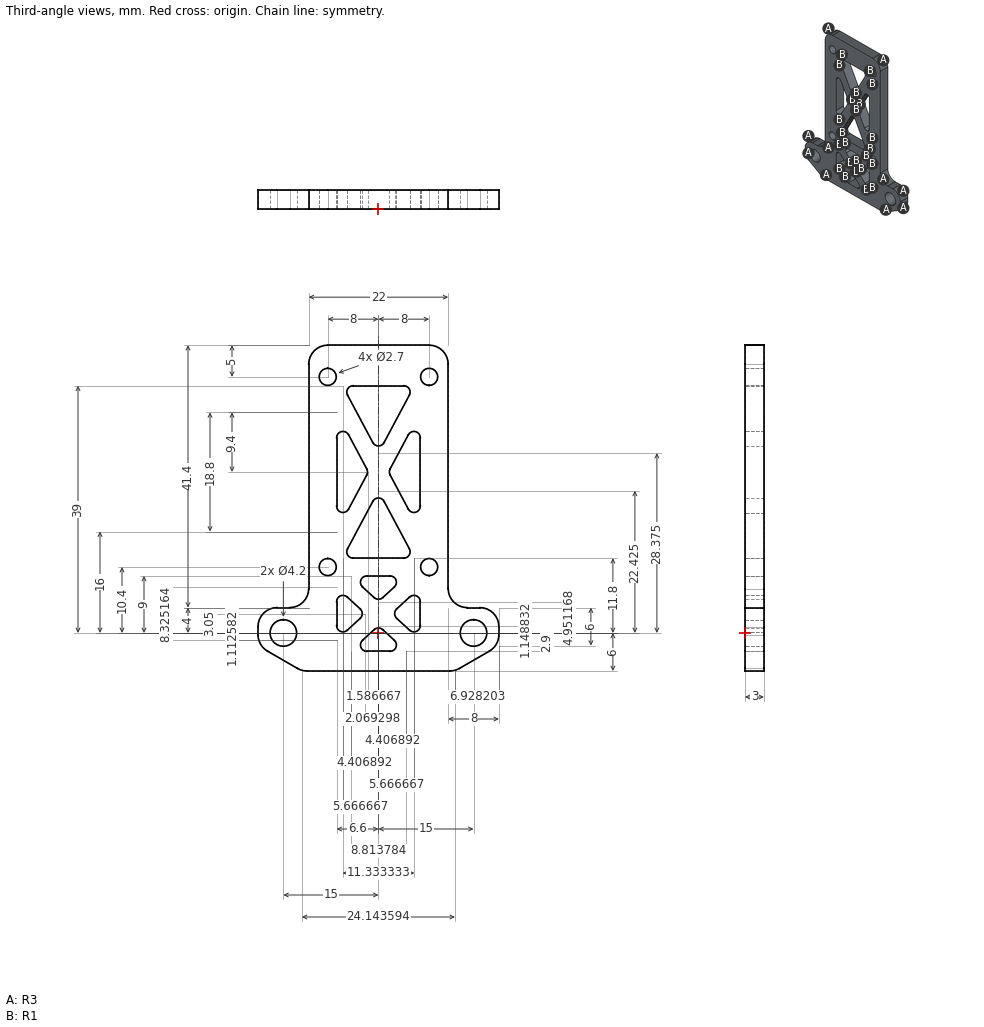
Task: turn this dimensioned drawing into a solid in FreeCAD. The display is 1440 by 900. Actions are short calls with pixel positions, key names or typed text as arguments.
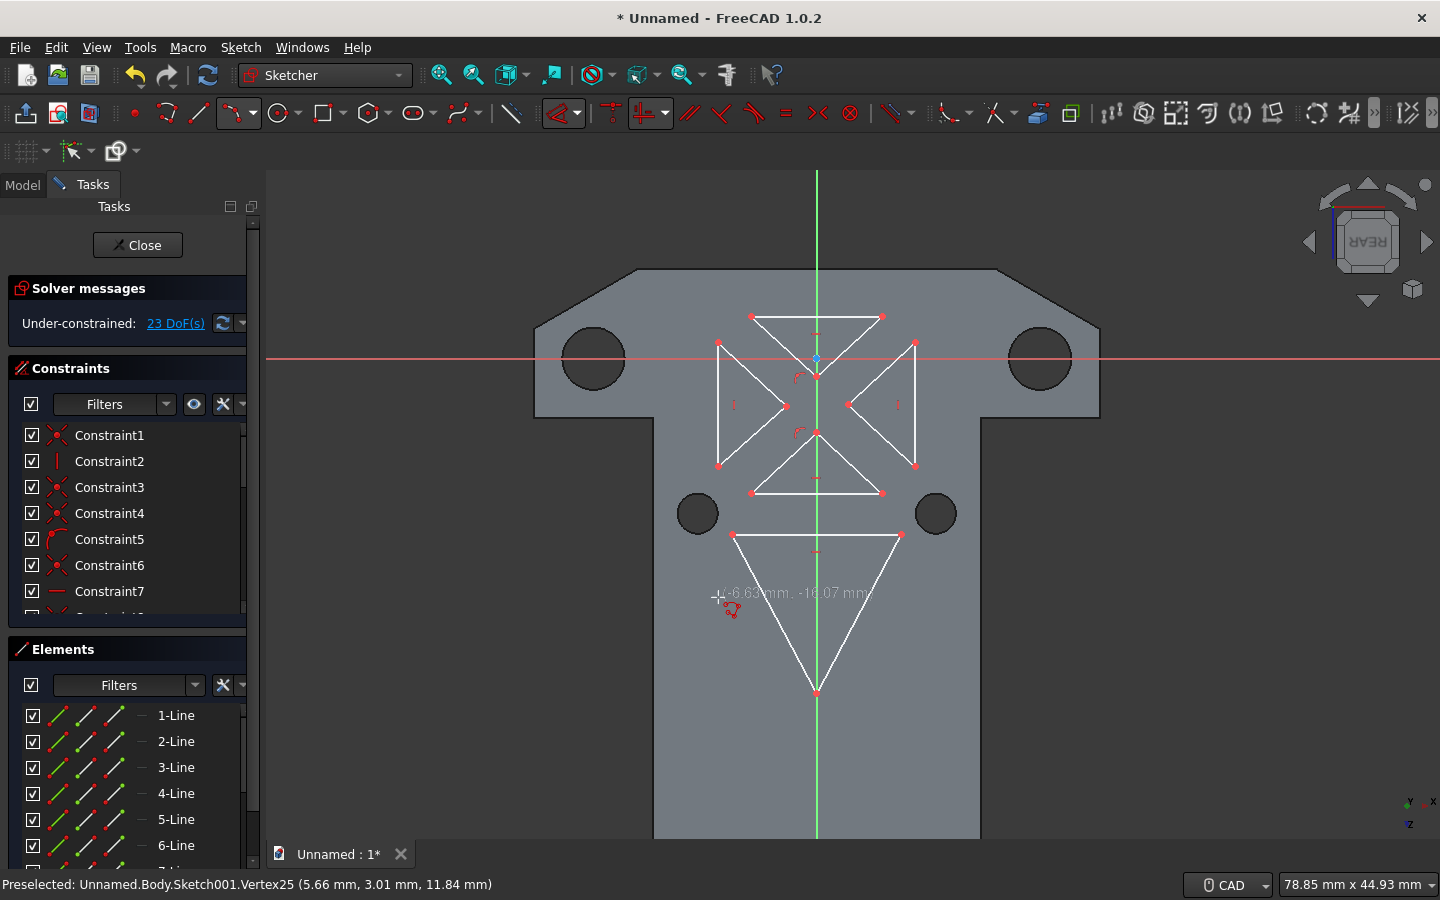
scroll(719, 255, down, 2)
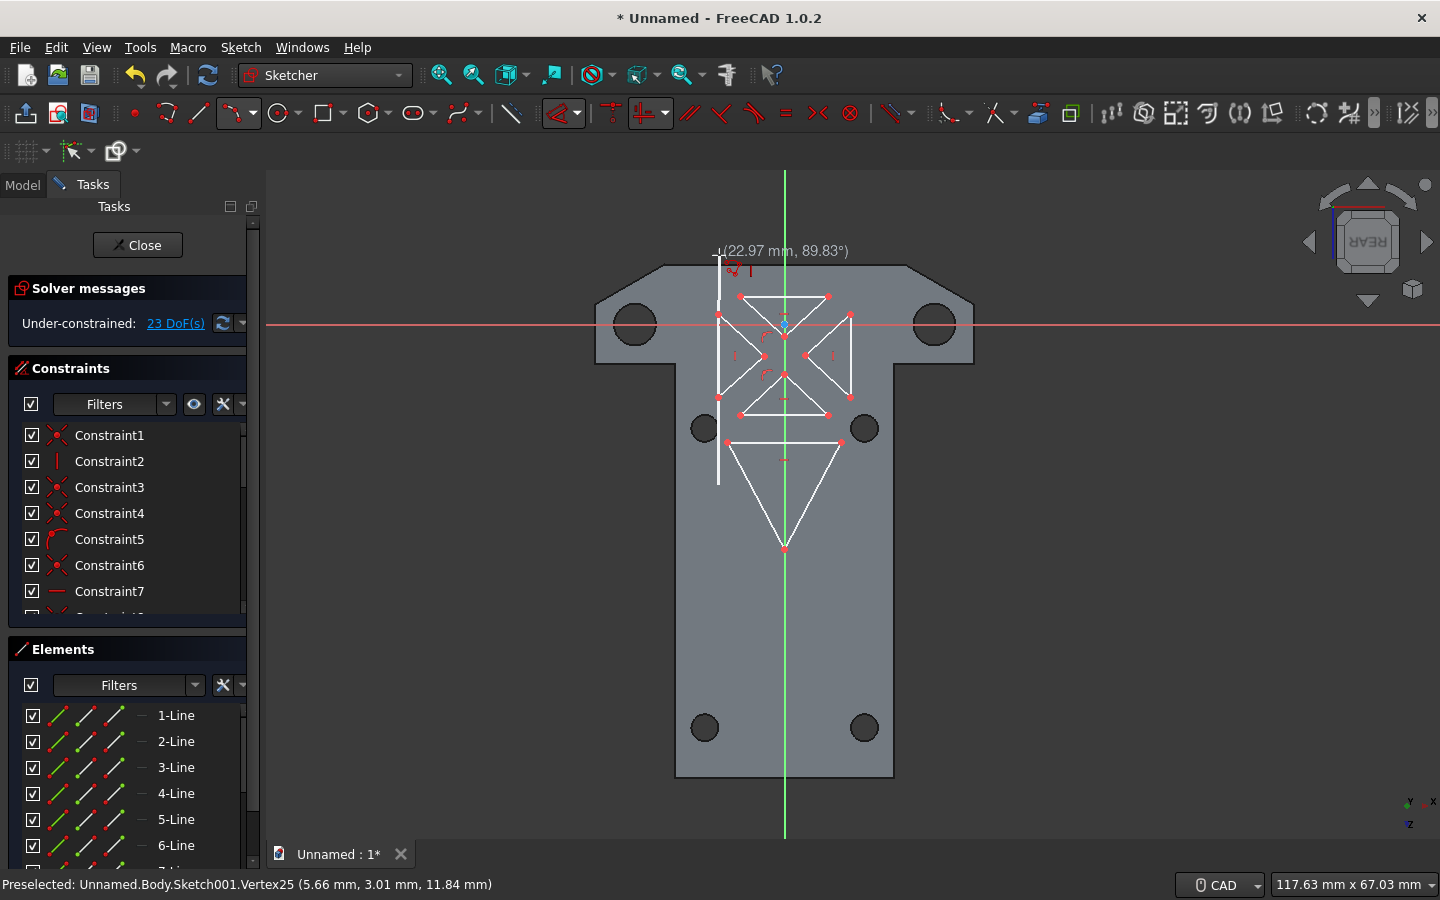
click(718, 672)
click(769, 578)
click(718, 485)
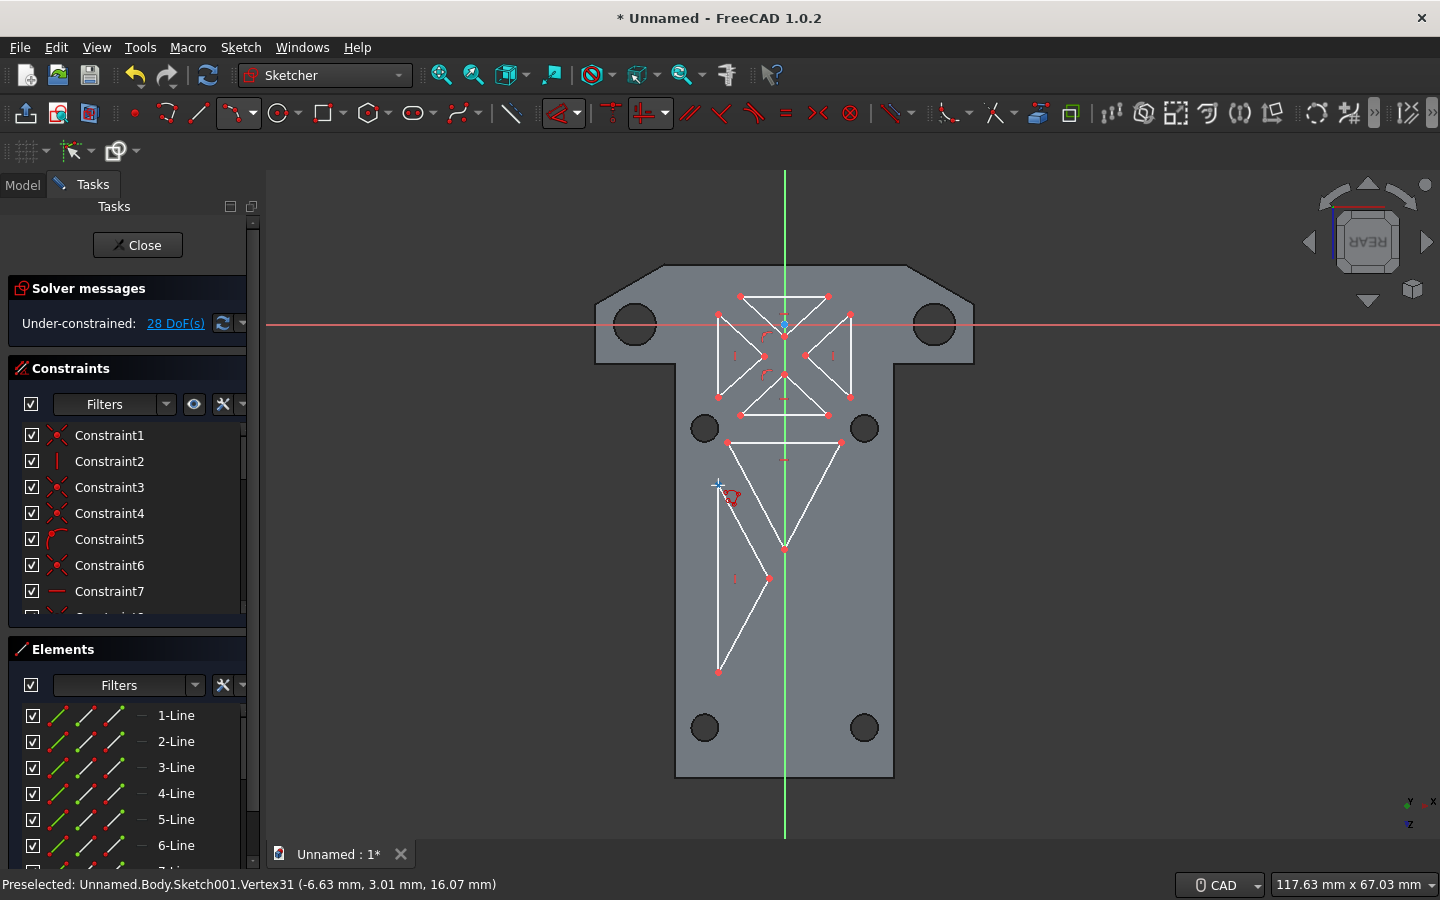
click(785, 608)
click(728, 714)
click(841, 714)
click(785, 609)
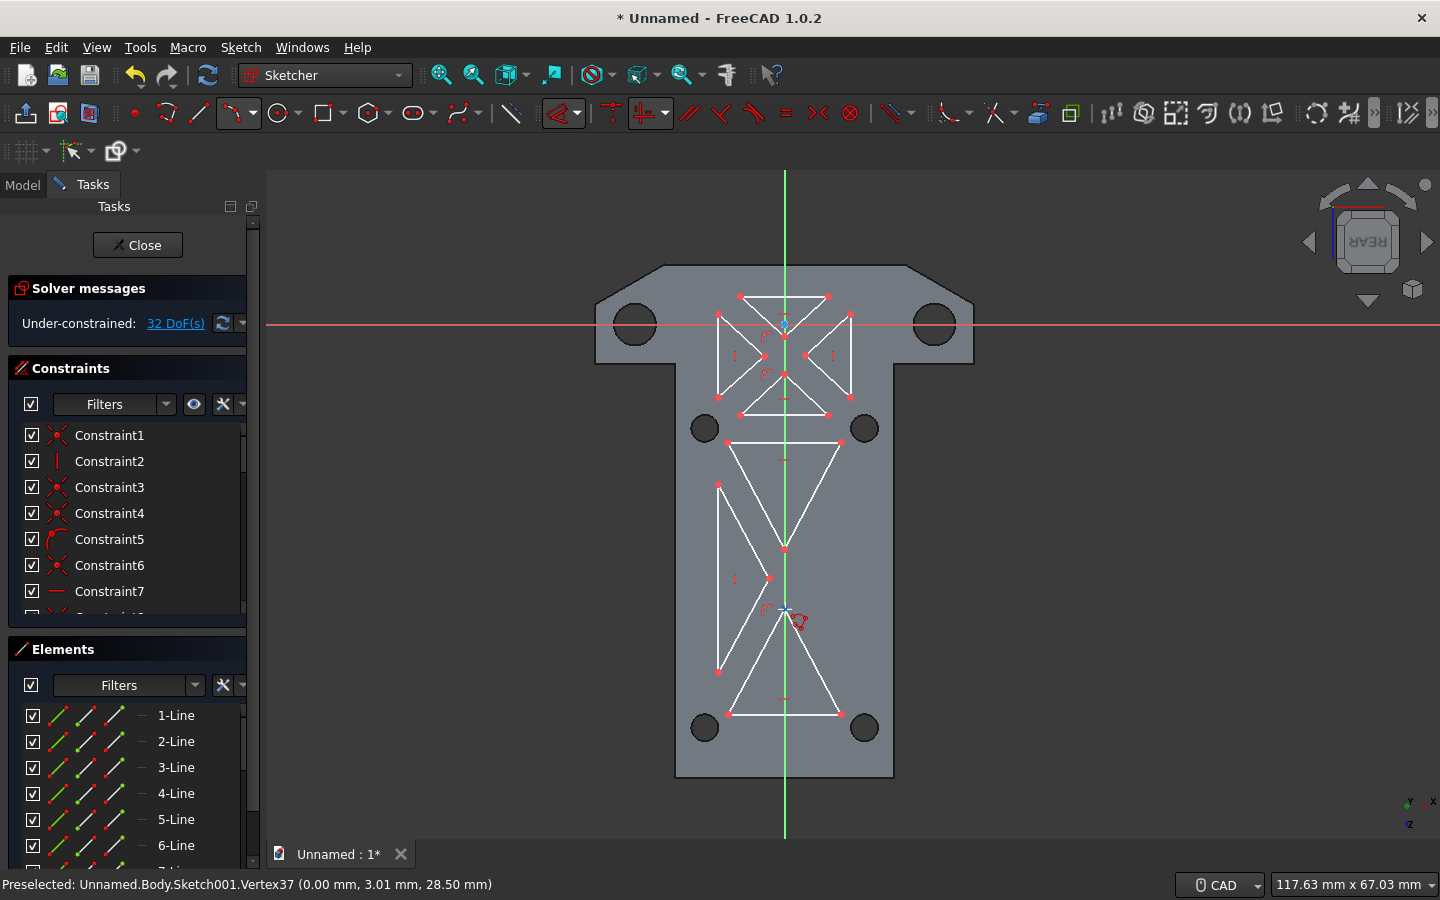
click(851, 484)
click(800, 578)
click(851, 672)
click(851, 485)
key(Escape)
key(Escape)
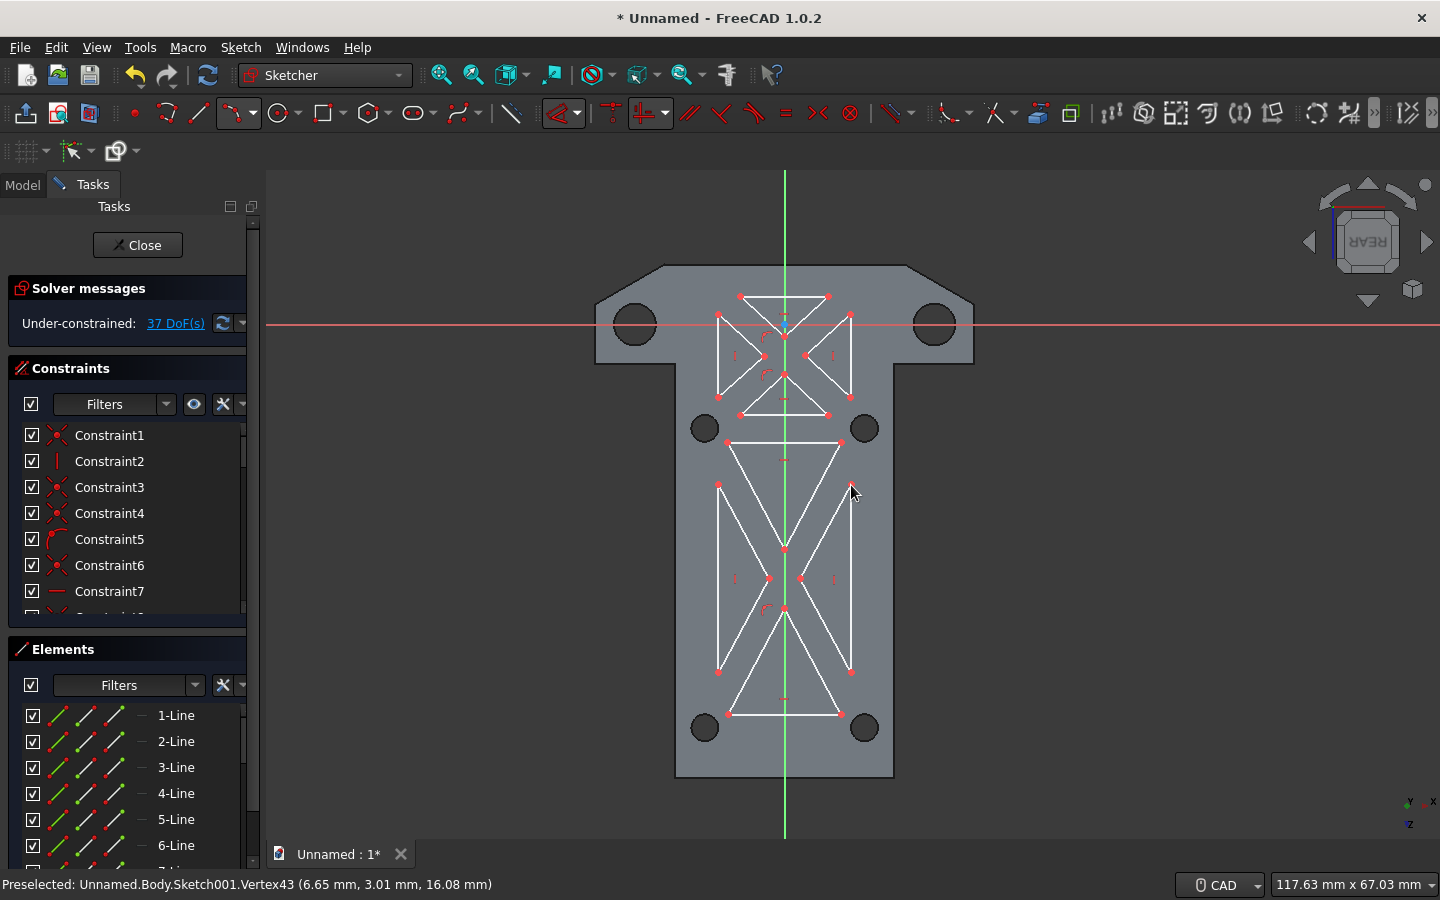
click(764, 356)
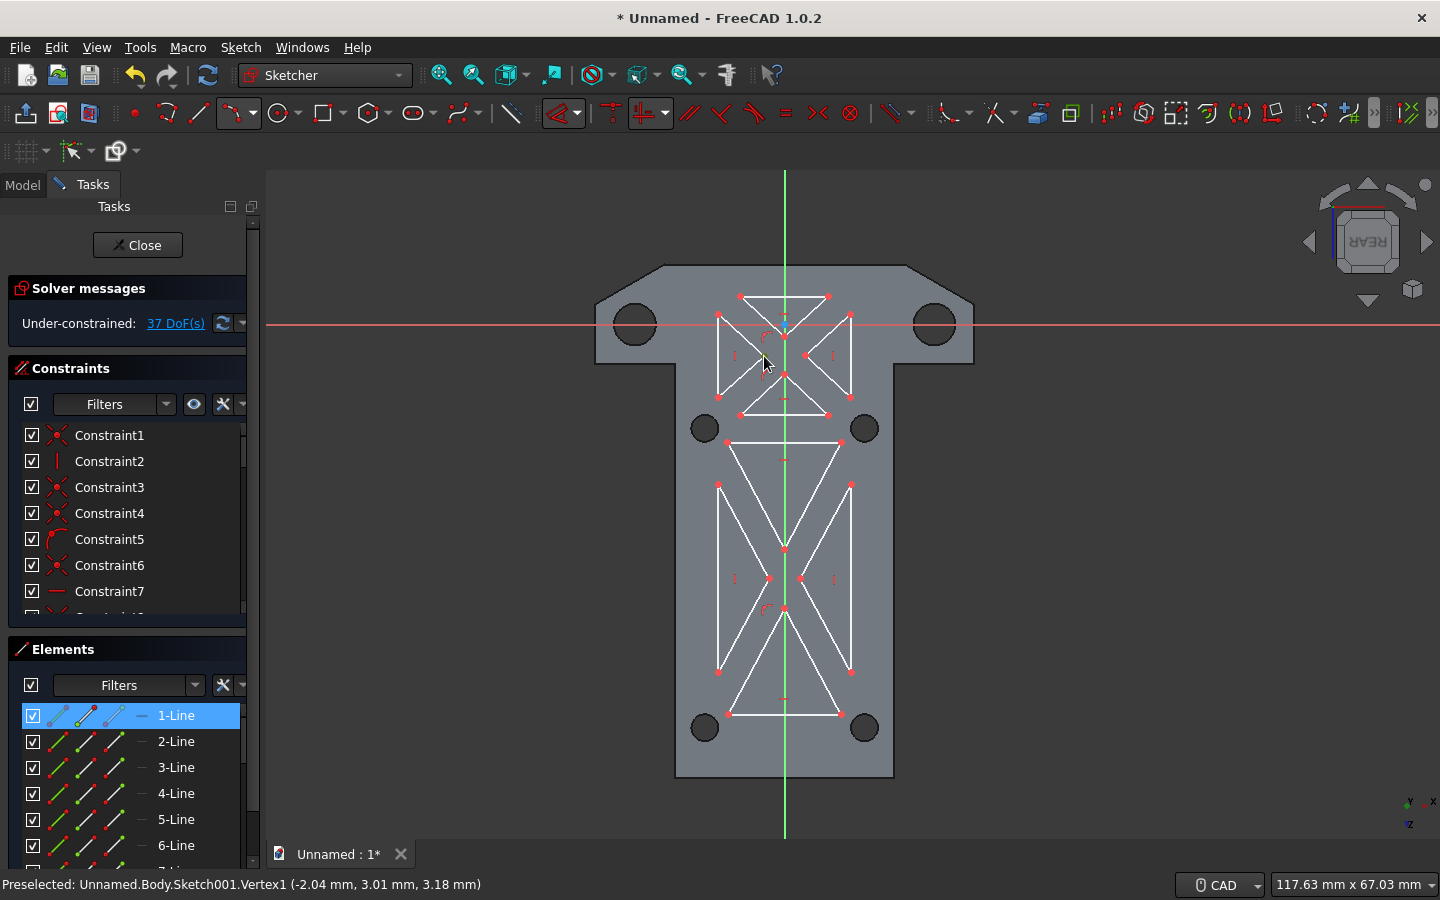
click(806, 356)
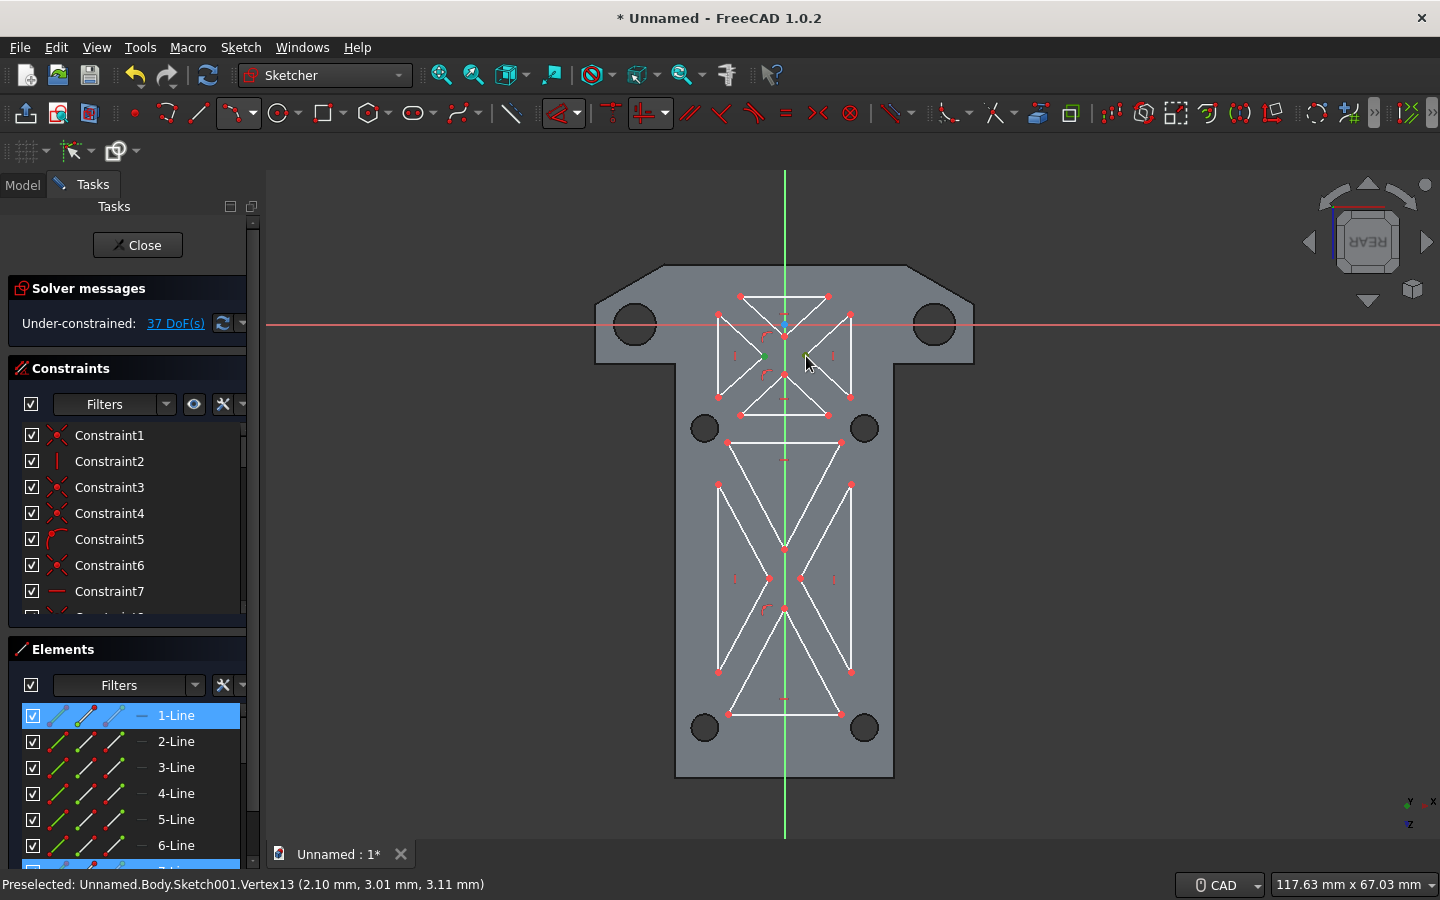
click(785, 767)